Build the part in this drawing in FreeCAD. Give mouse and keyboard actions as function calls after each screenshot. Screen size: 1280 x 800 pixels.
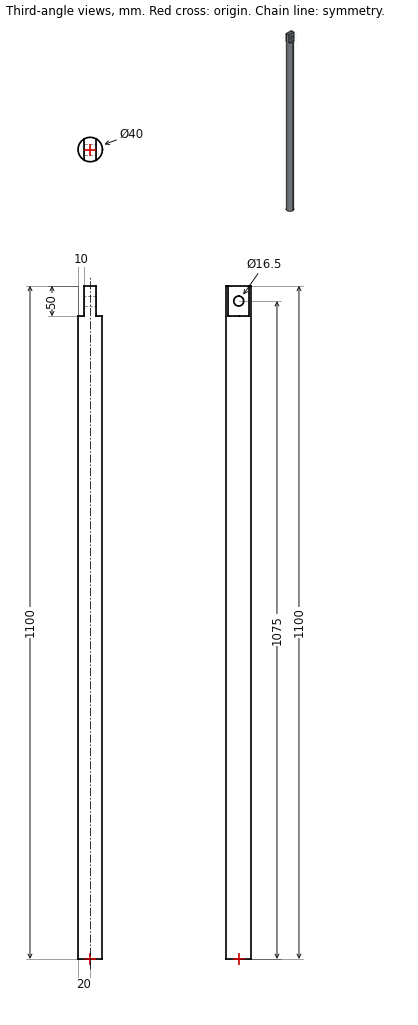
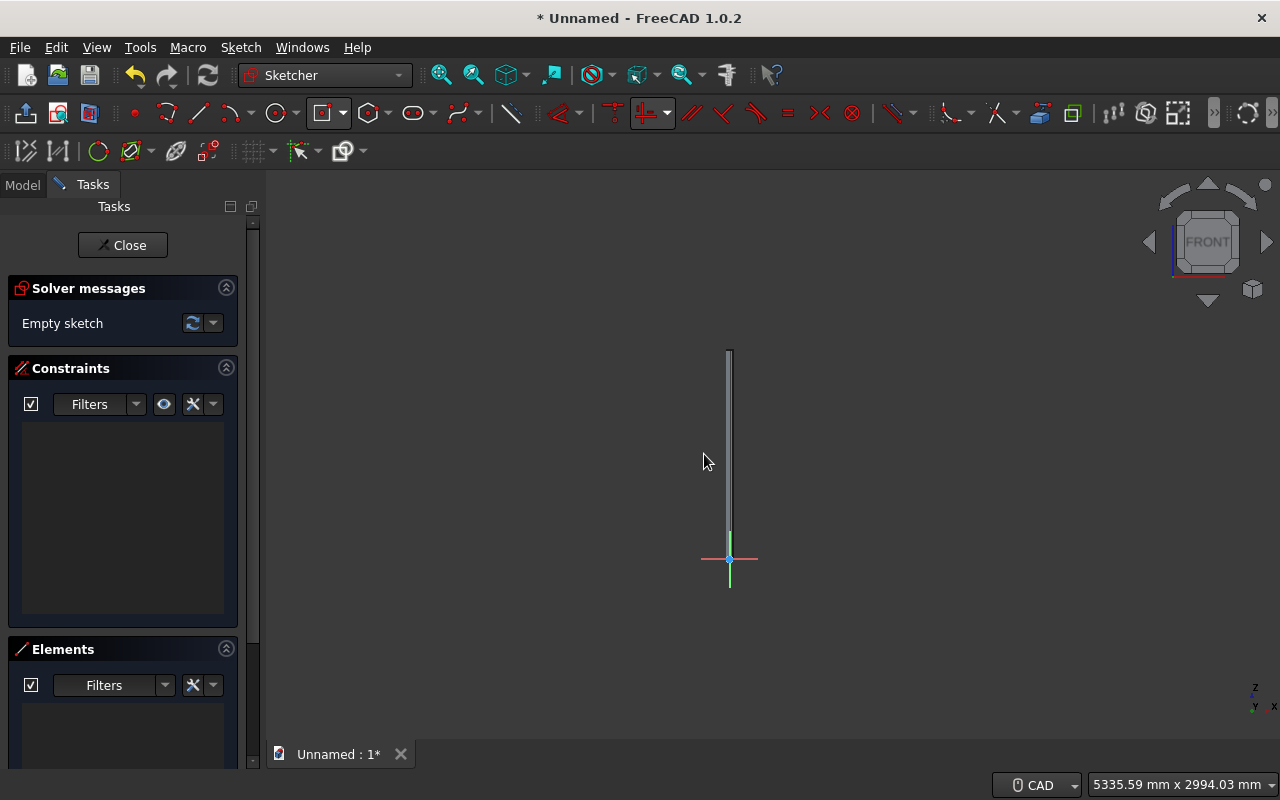
scroll(731, 349, up, 15)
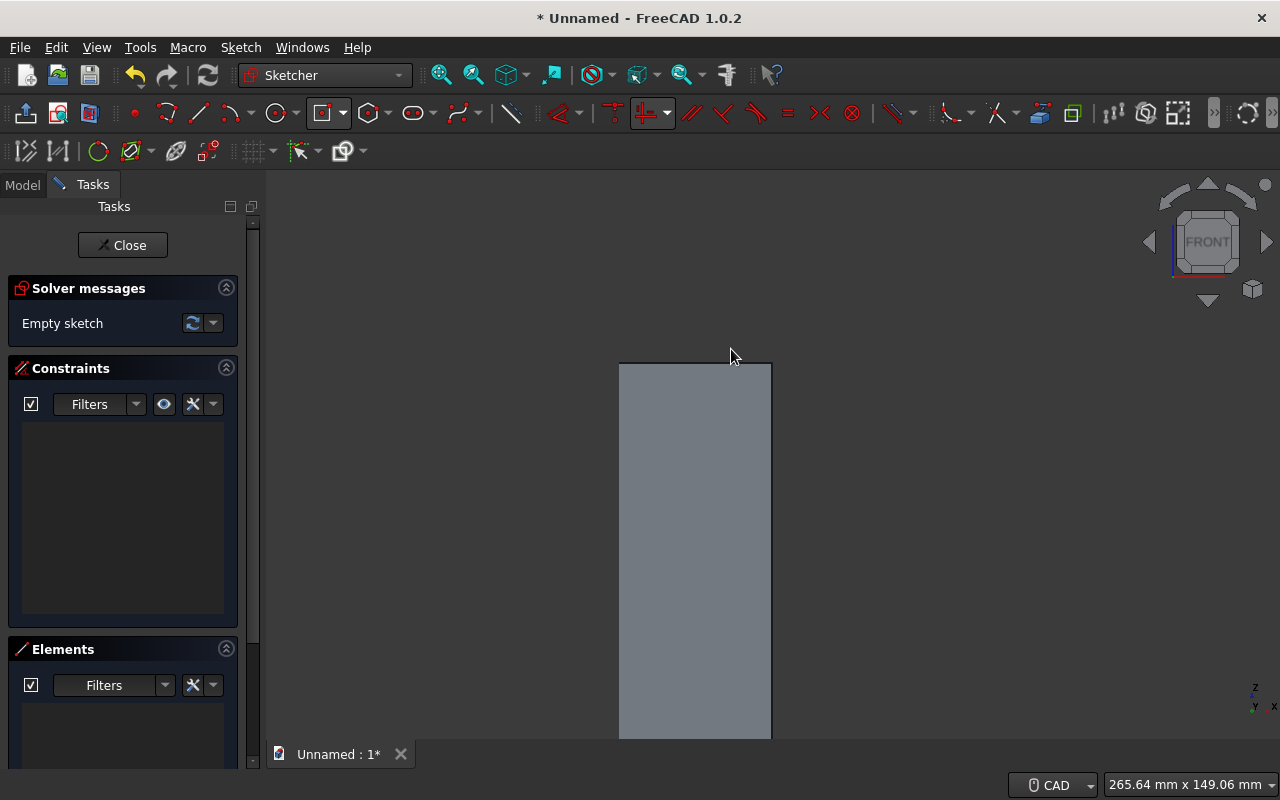
scroll(684, 462, up, 3)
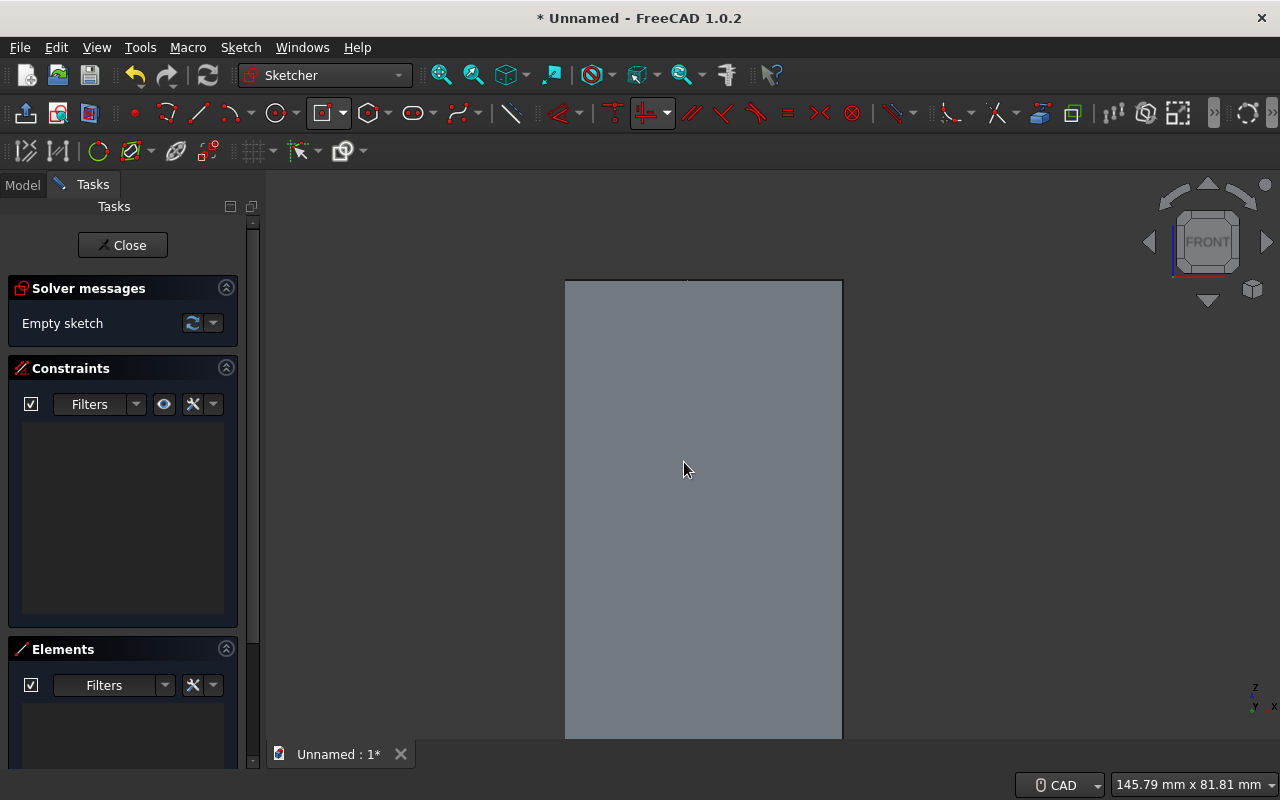
key(g)
key(r)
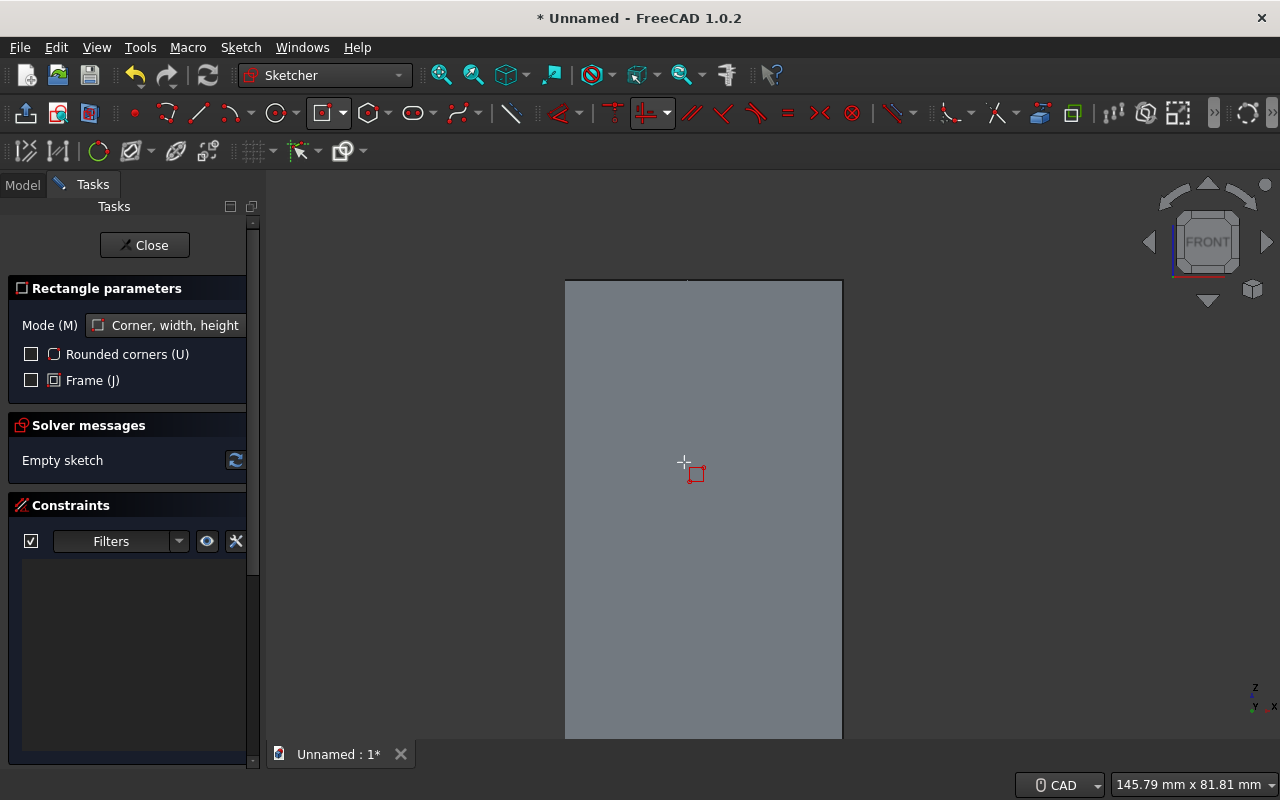
click(565, 280)
click(635, 628)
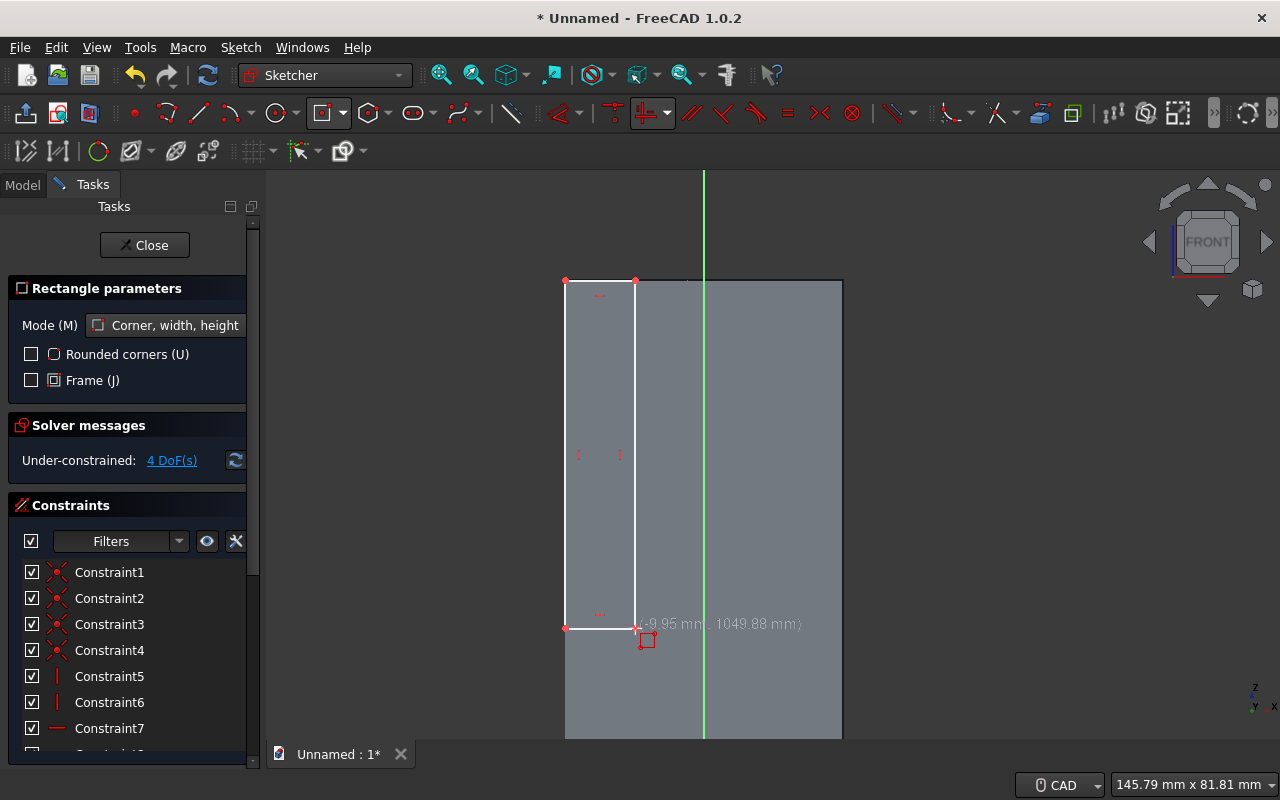
click(774, 280)
click(843, 628)
key(Escape)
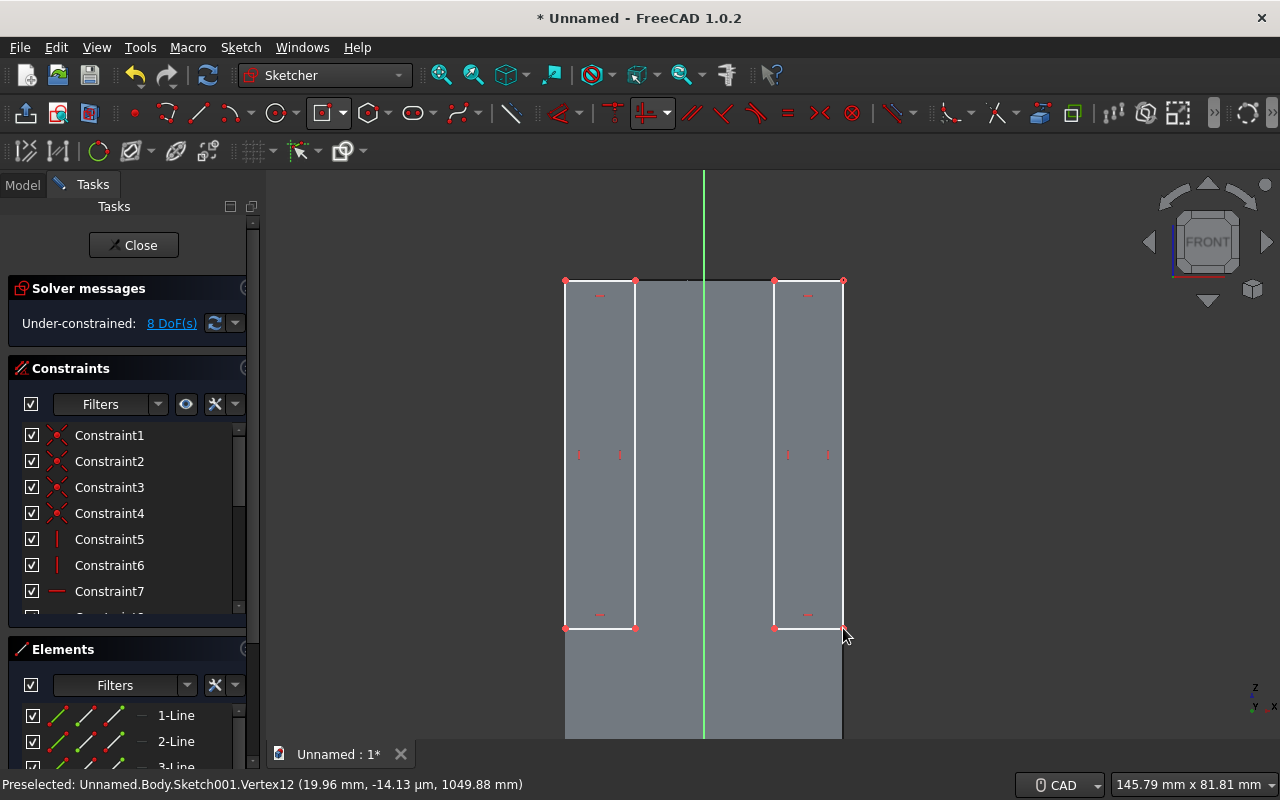
click(635, 281)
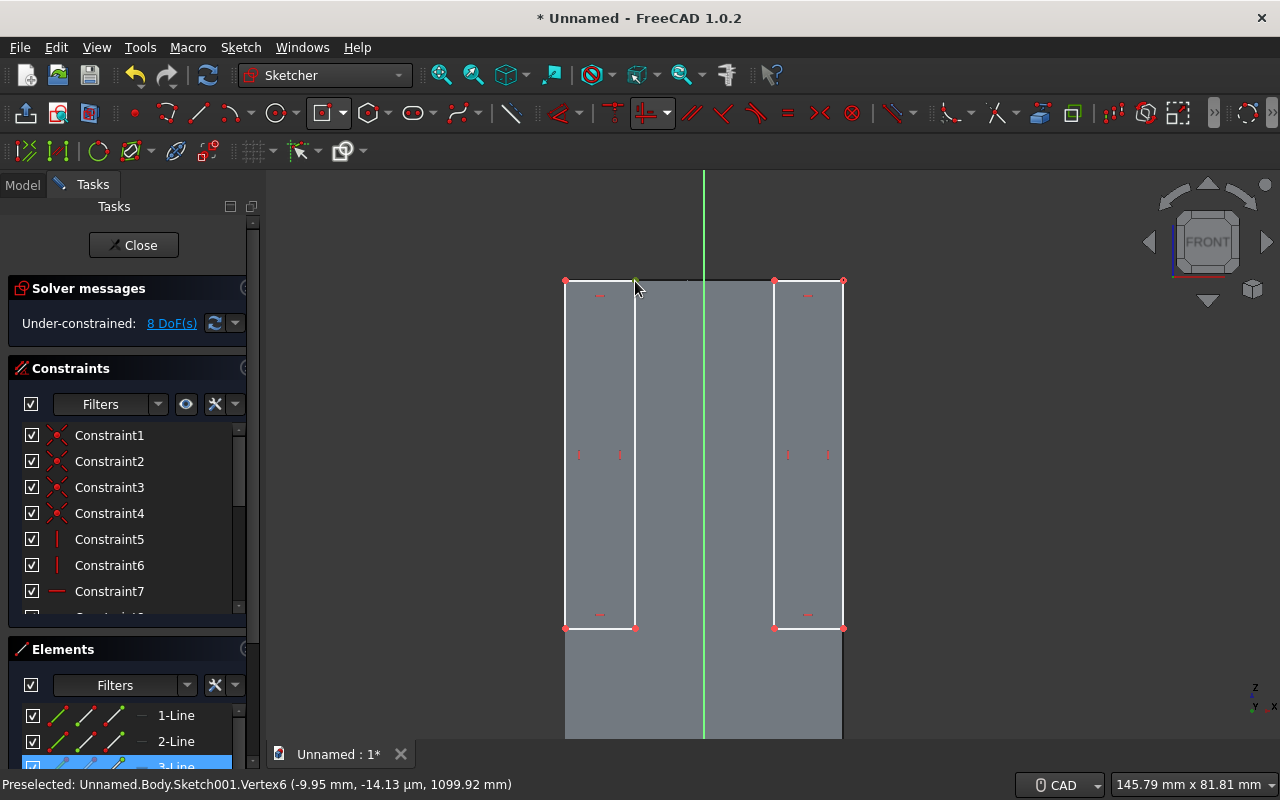
click(774, 281)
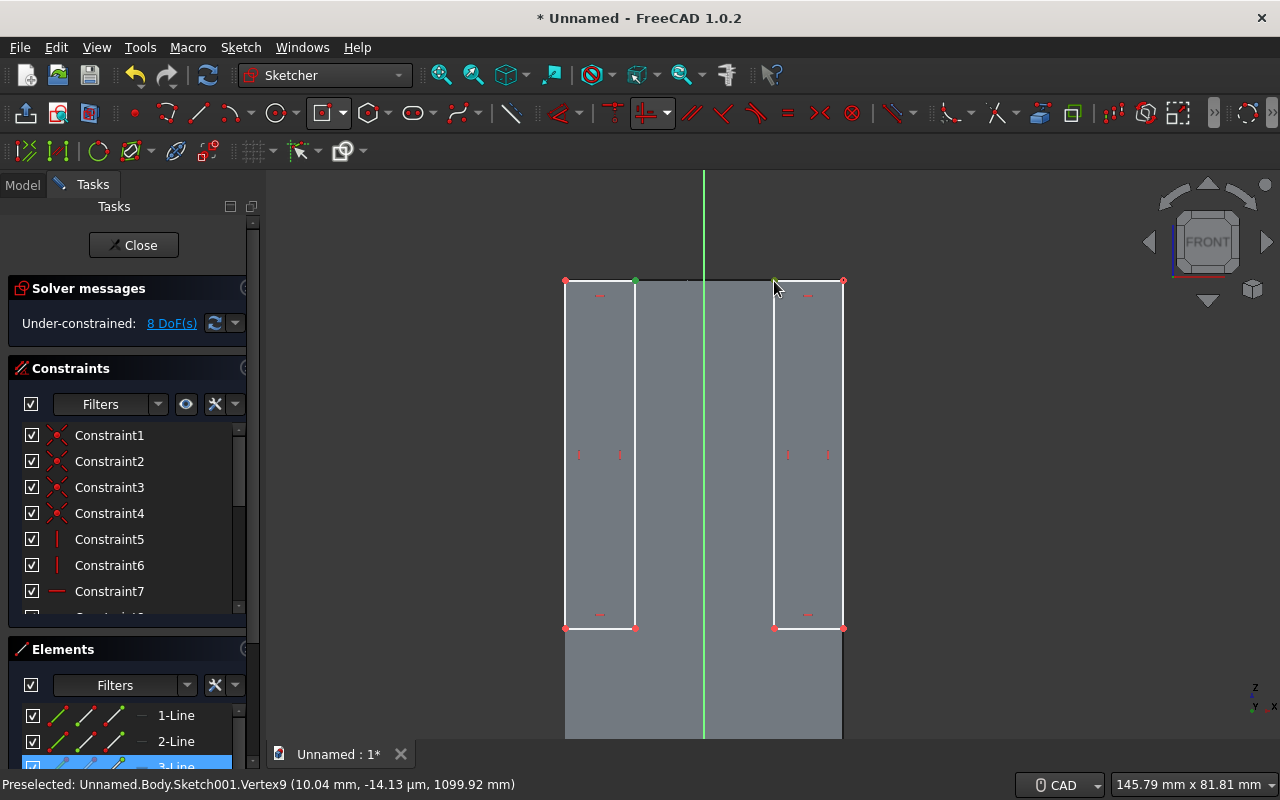
click(704, 674)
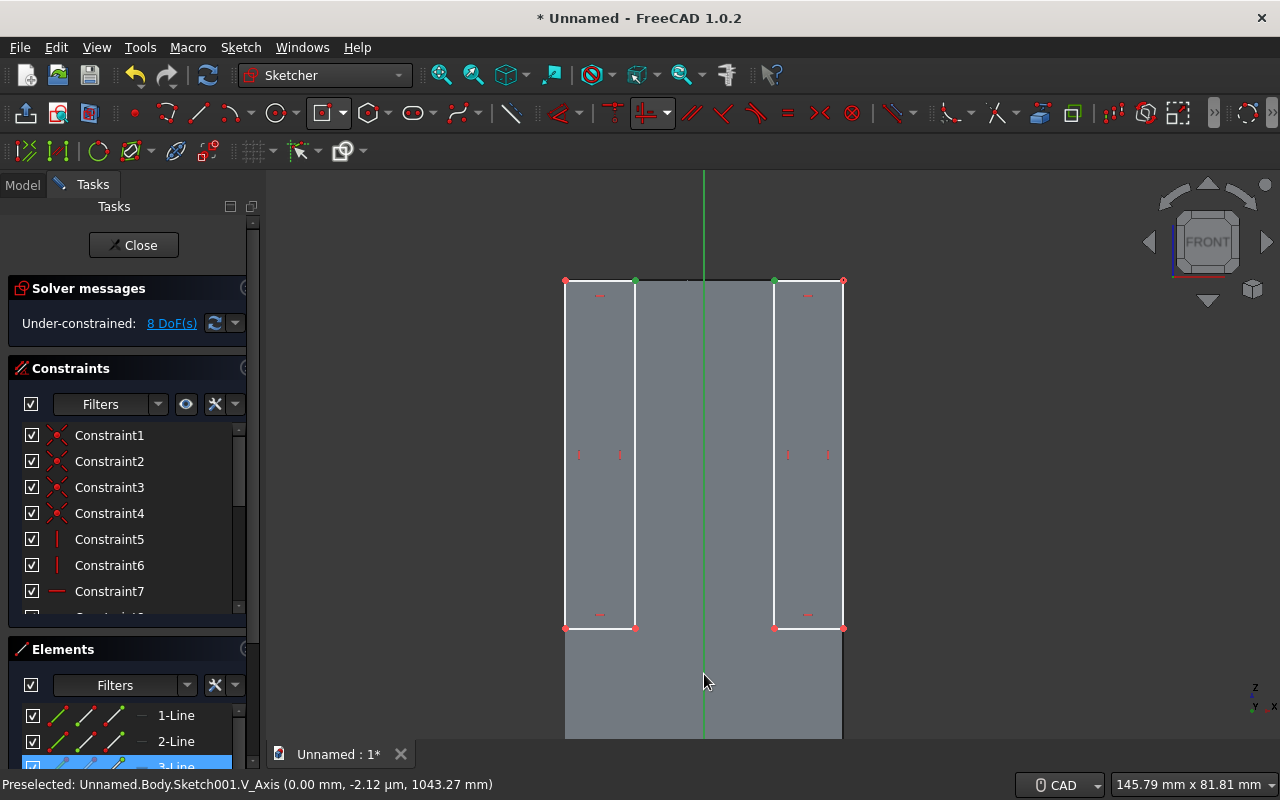
click(820, 114)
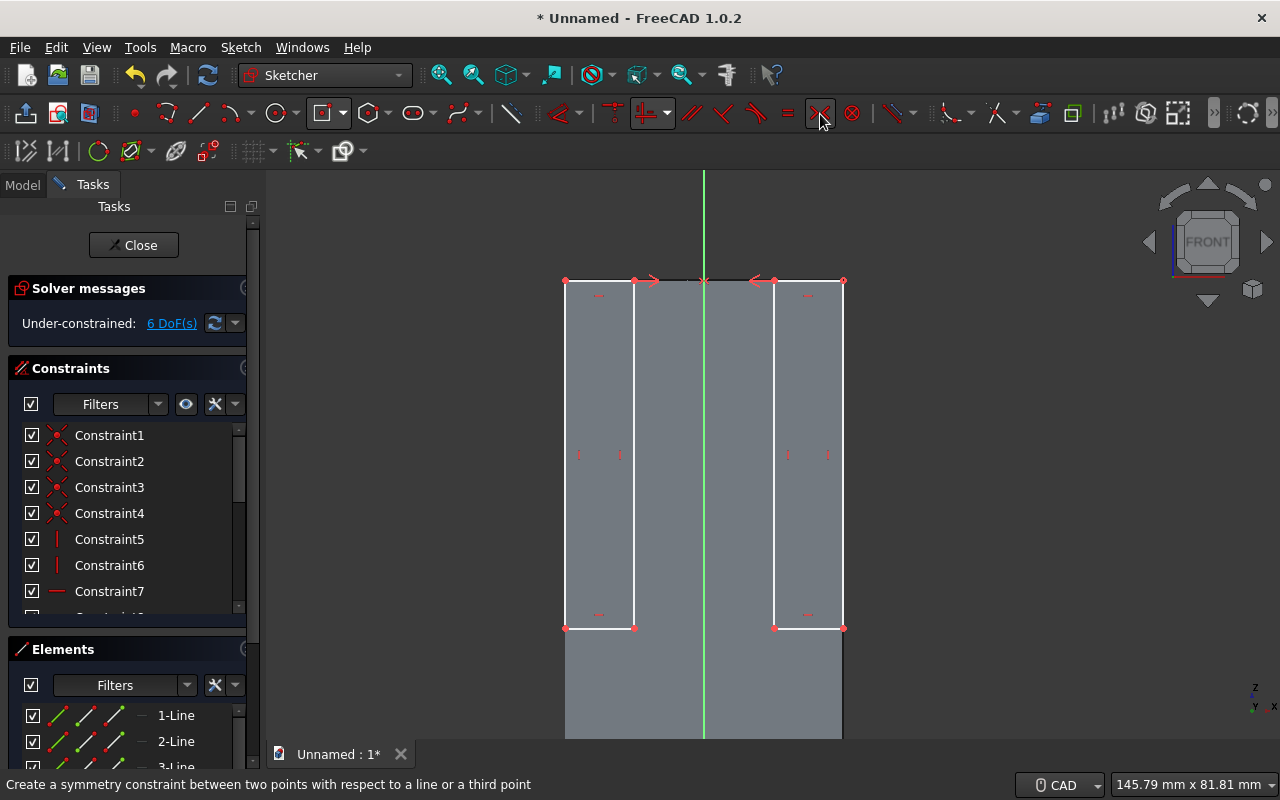
click(565, 629)